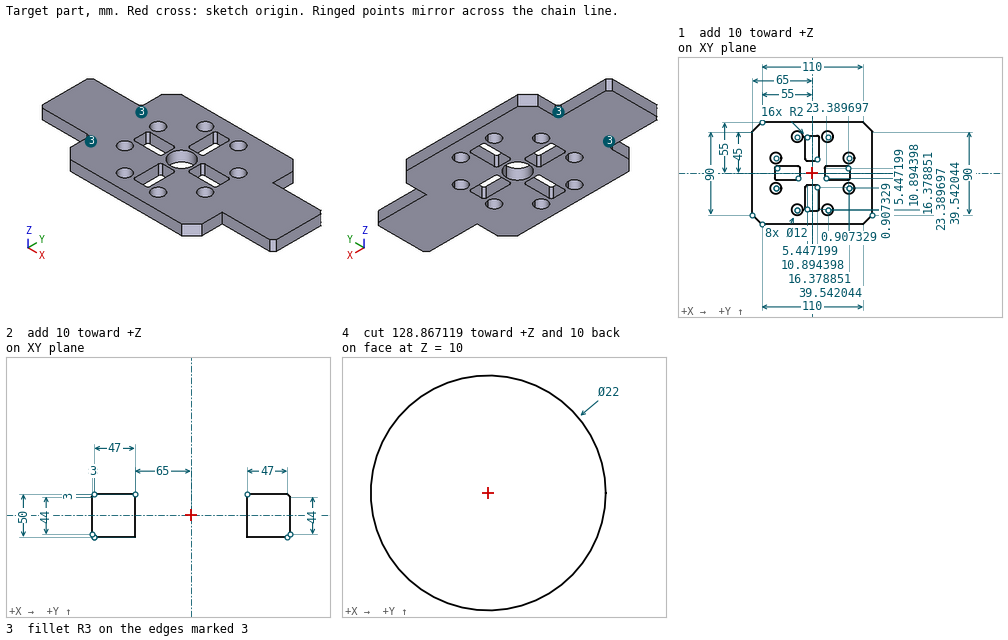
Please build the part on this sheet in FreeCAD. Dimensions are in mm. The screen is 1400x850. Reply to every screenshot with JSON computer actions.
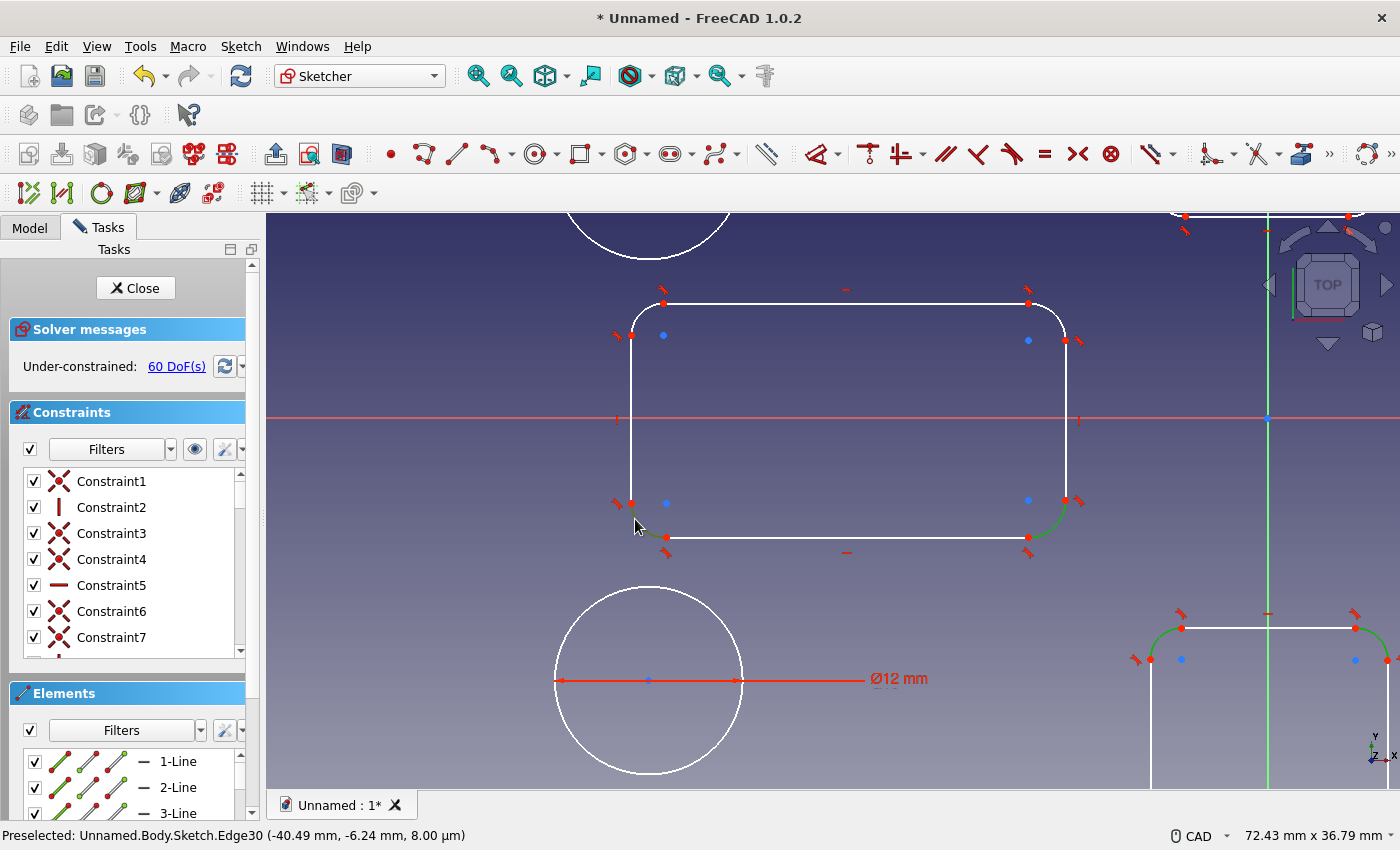
{"action": "left_click", "coordinate": [649, 307]}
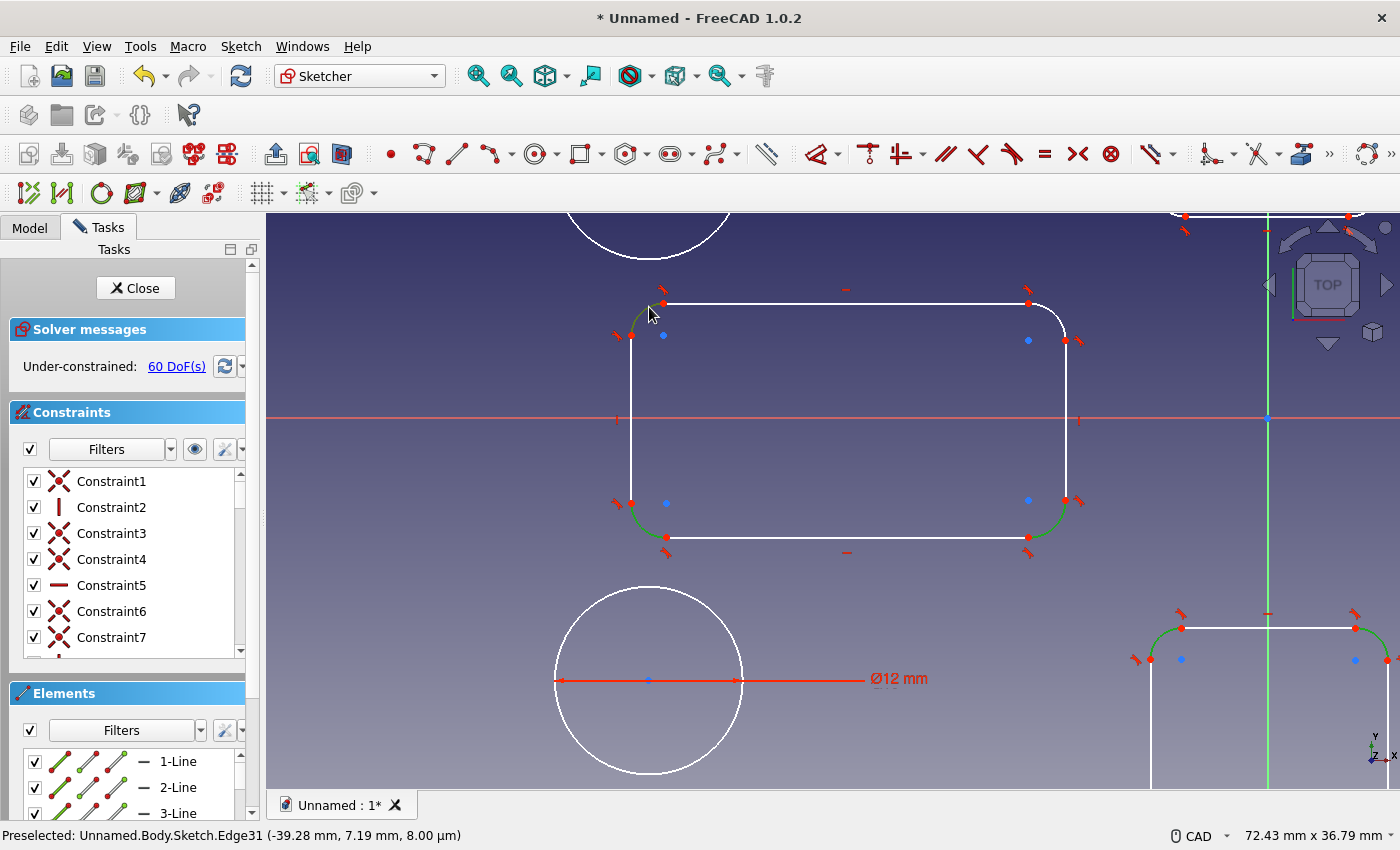
{"action": "left_click", "coordinate": [1062, 324]}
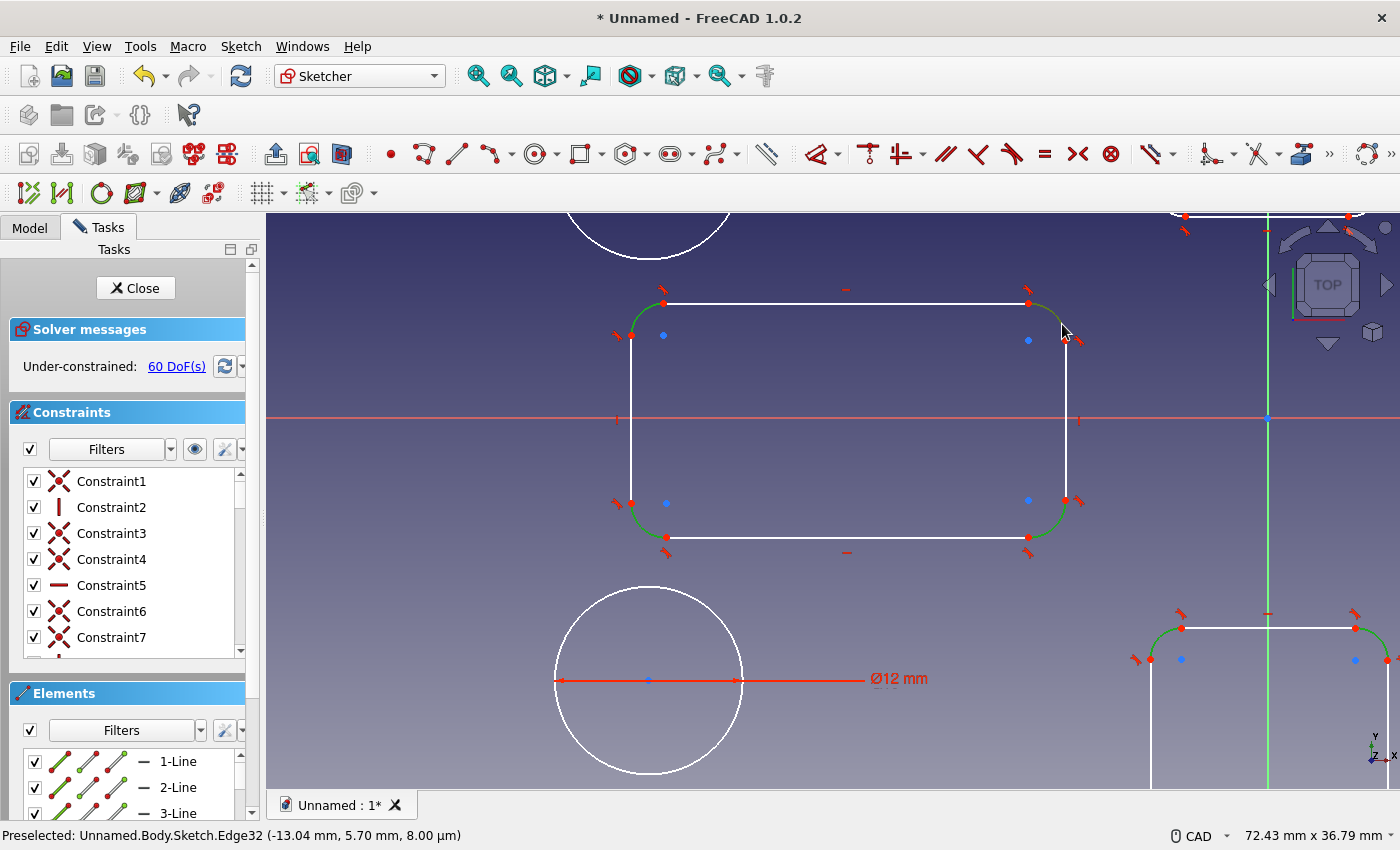
{"action": "scroll", "coordinate": [637, 522], "scroll_direction": "down", "scroll_amount": 8}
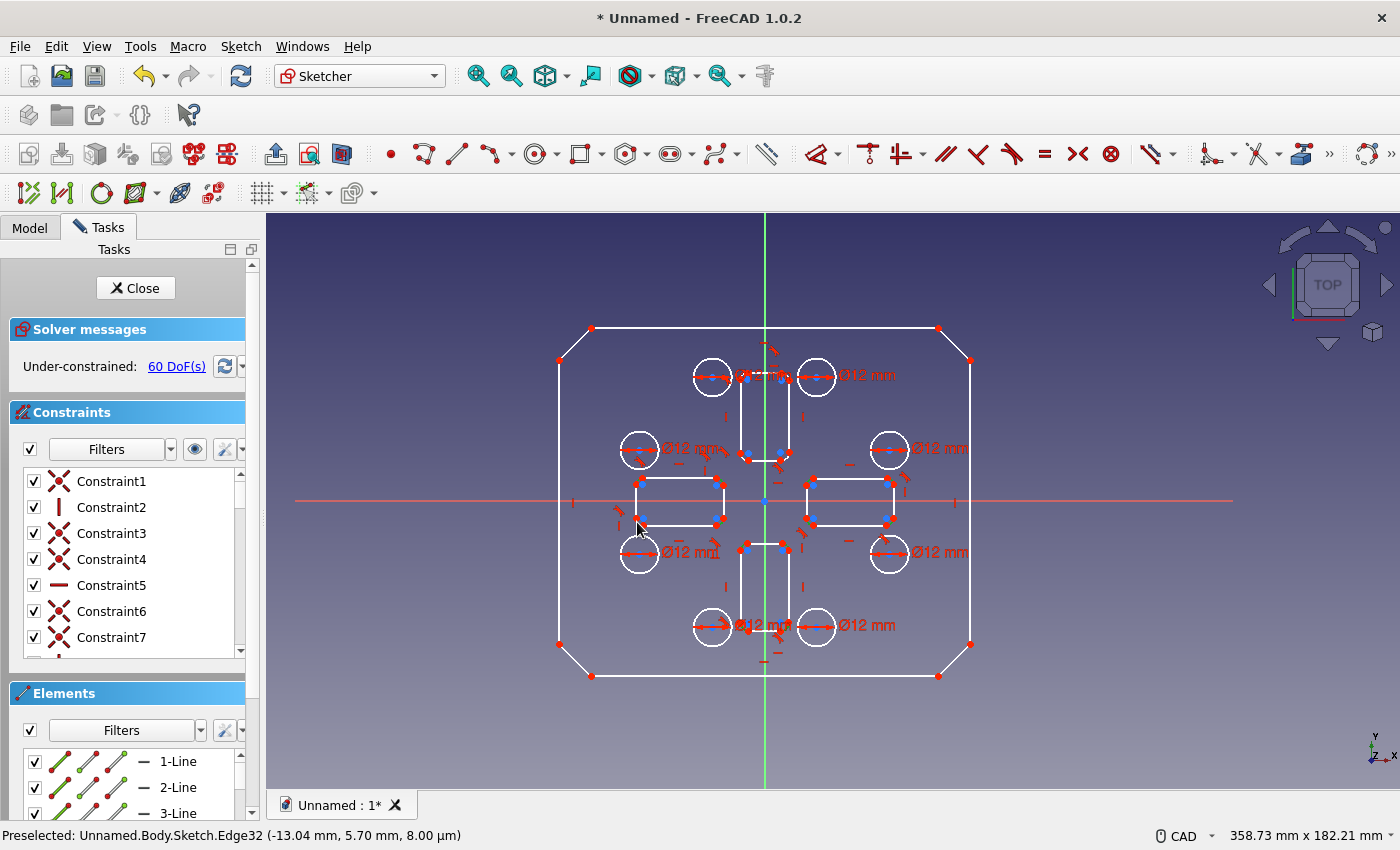
{"action": "scroll", "coordinate": [785, 460], "scroll_direction": "up", "scroll_amount": 7}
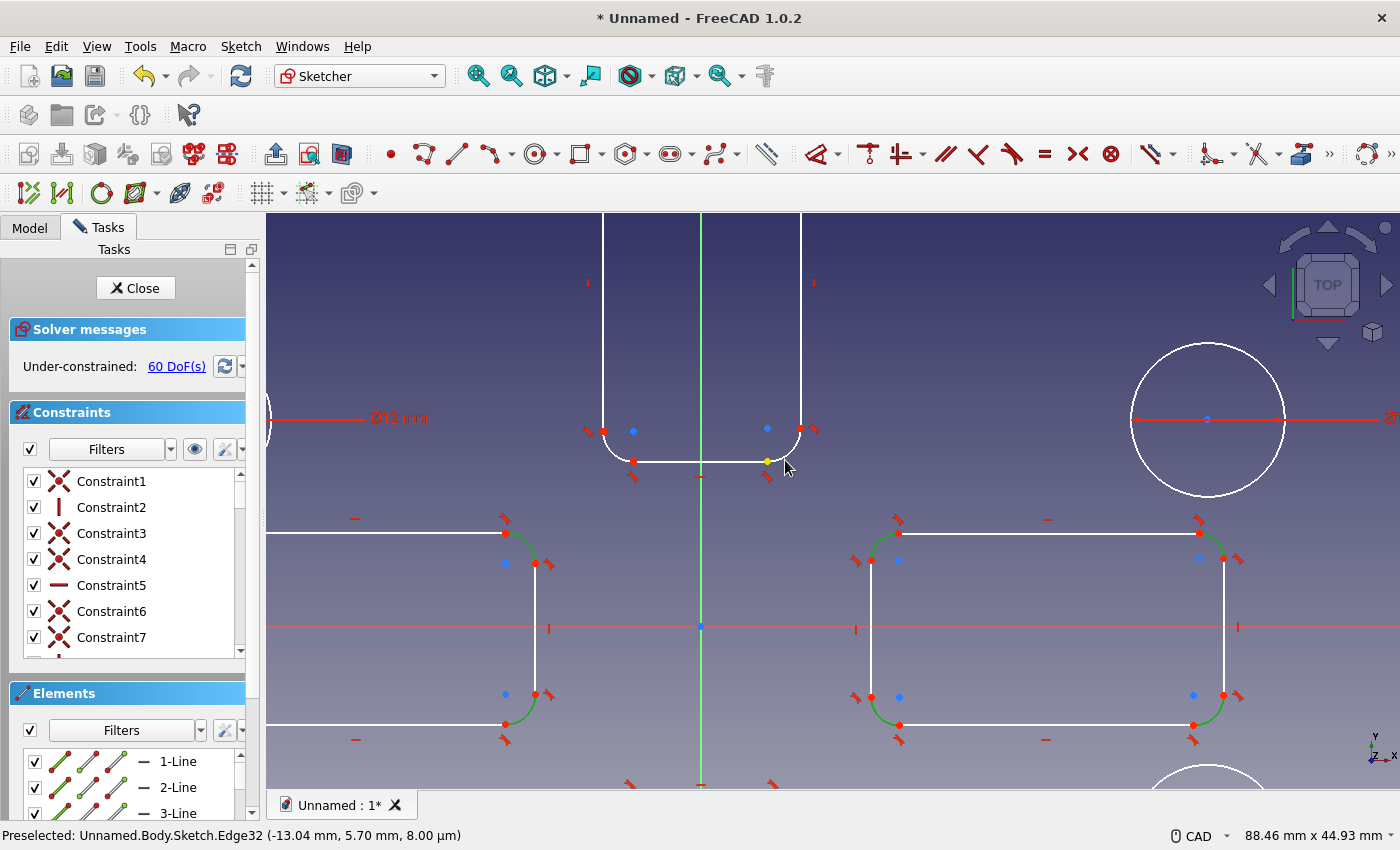
{"action": "left_click", "coordinate": [782, 458]}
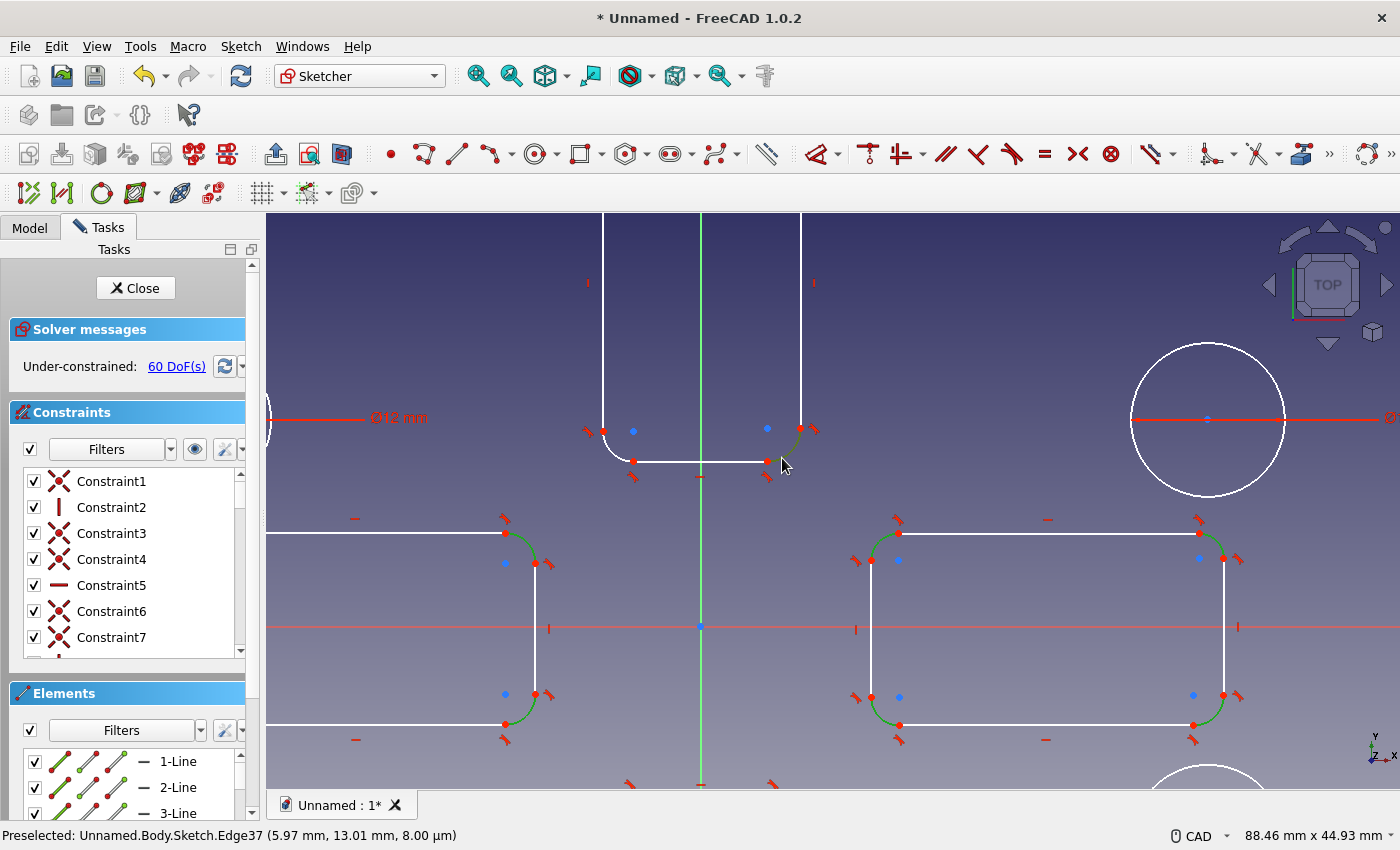
{"action": "left_click", "coordinate": [607, 445]}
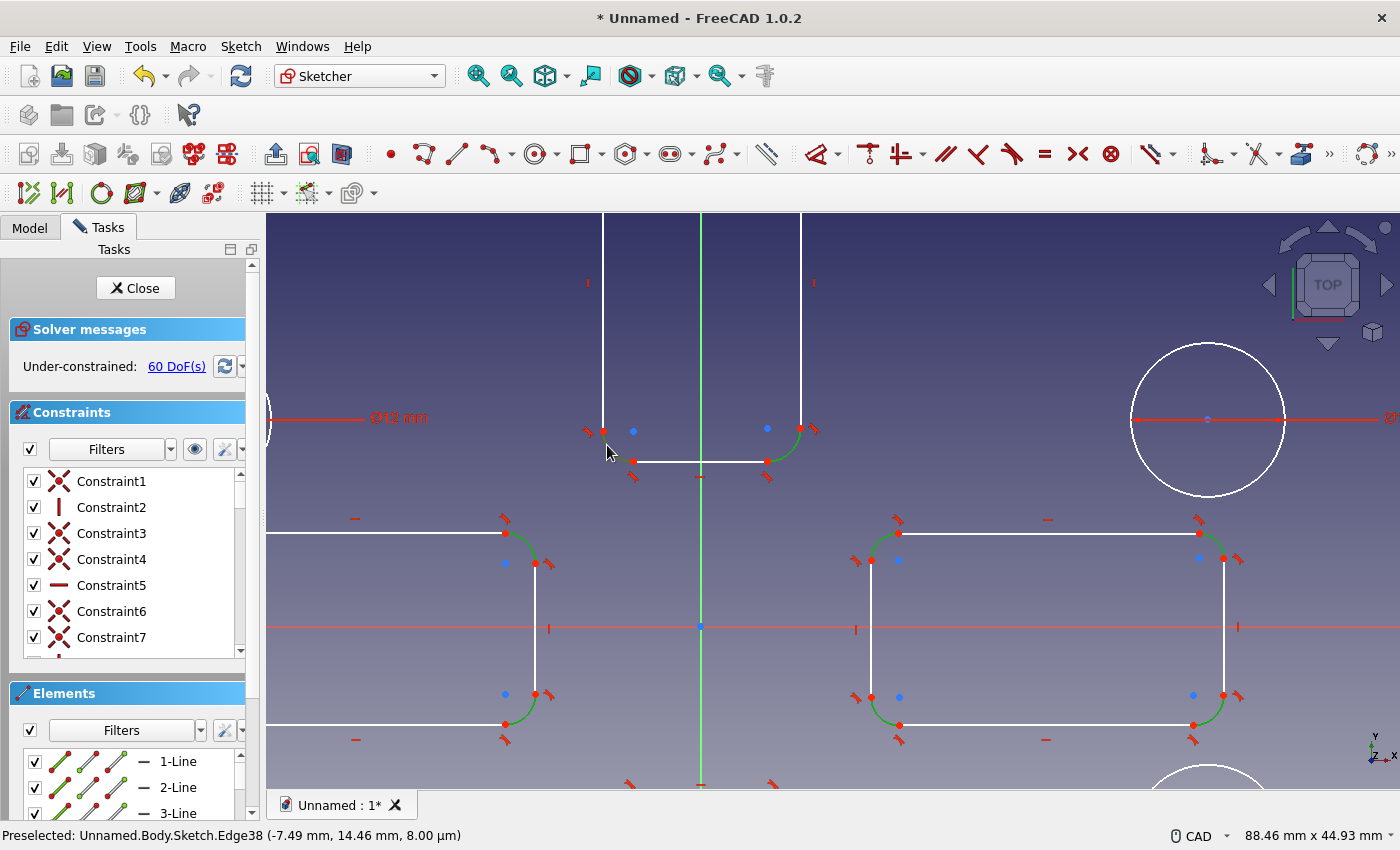
{"action": "scroll", "coordinate": [785, 460], "scroll_direction": "down", "scroll_amount": 7}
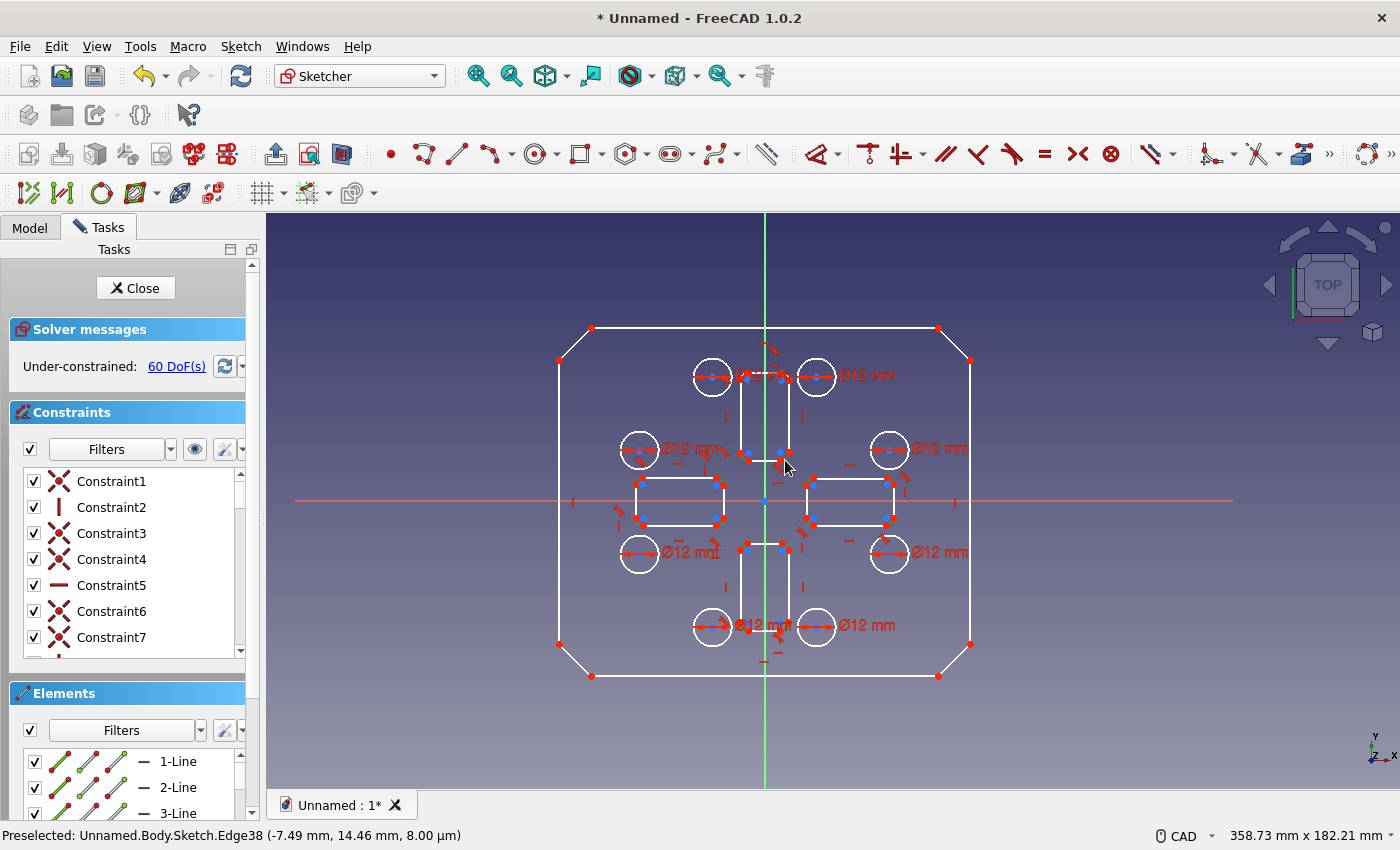
{"action": "scroll", "coordinate": [744, 374], "scroll_direction": "up", "scroll_amount": 8}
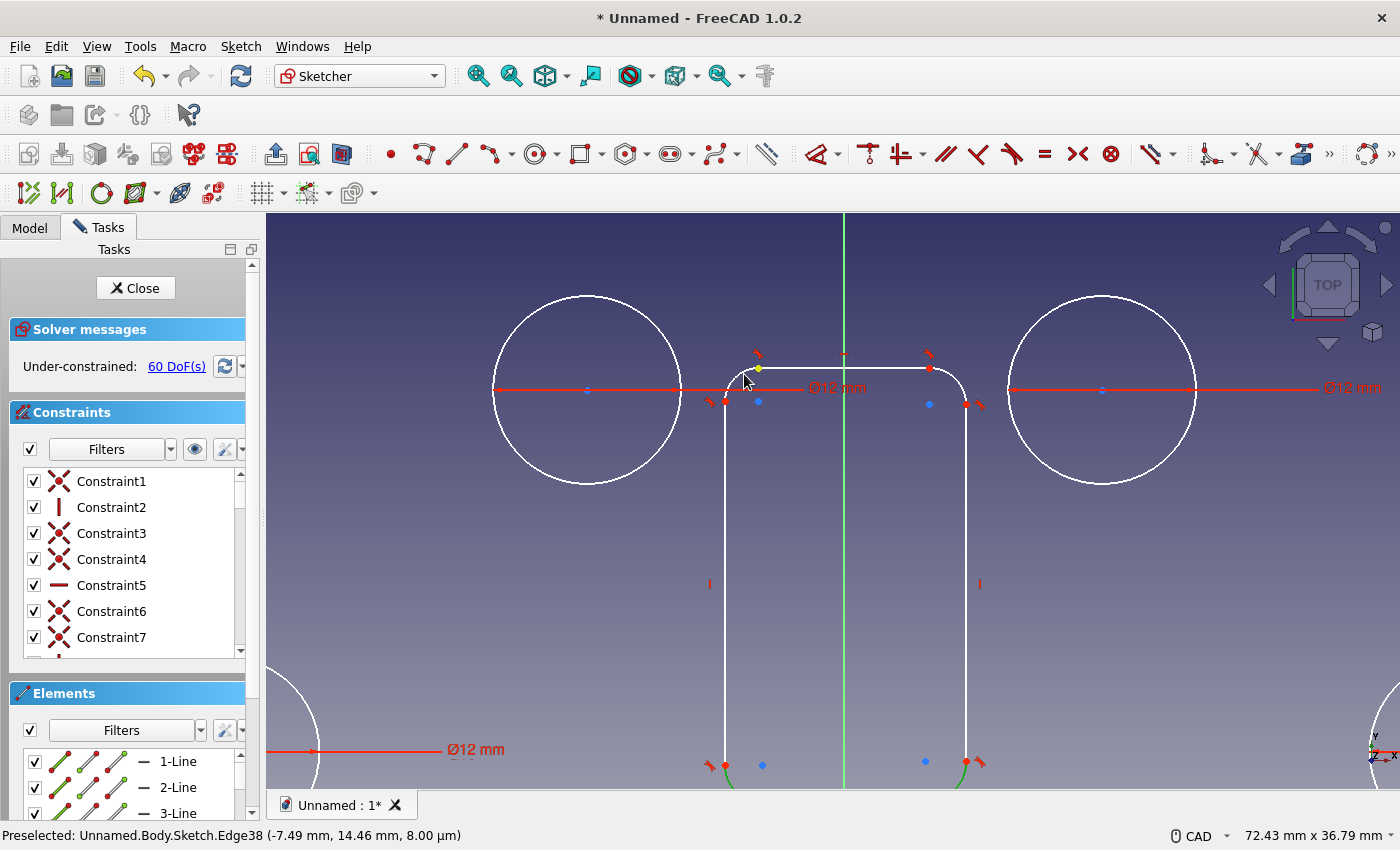
{"action": "left_click", "coordinate": [744, 372]}